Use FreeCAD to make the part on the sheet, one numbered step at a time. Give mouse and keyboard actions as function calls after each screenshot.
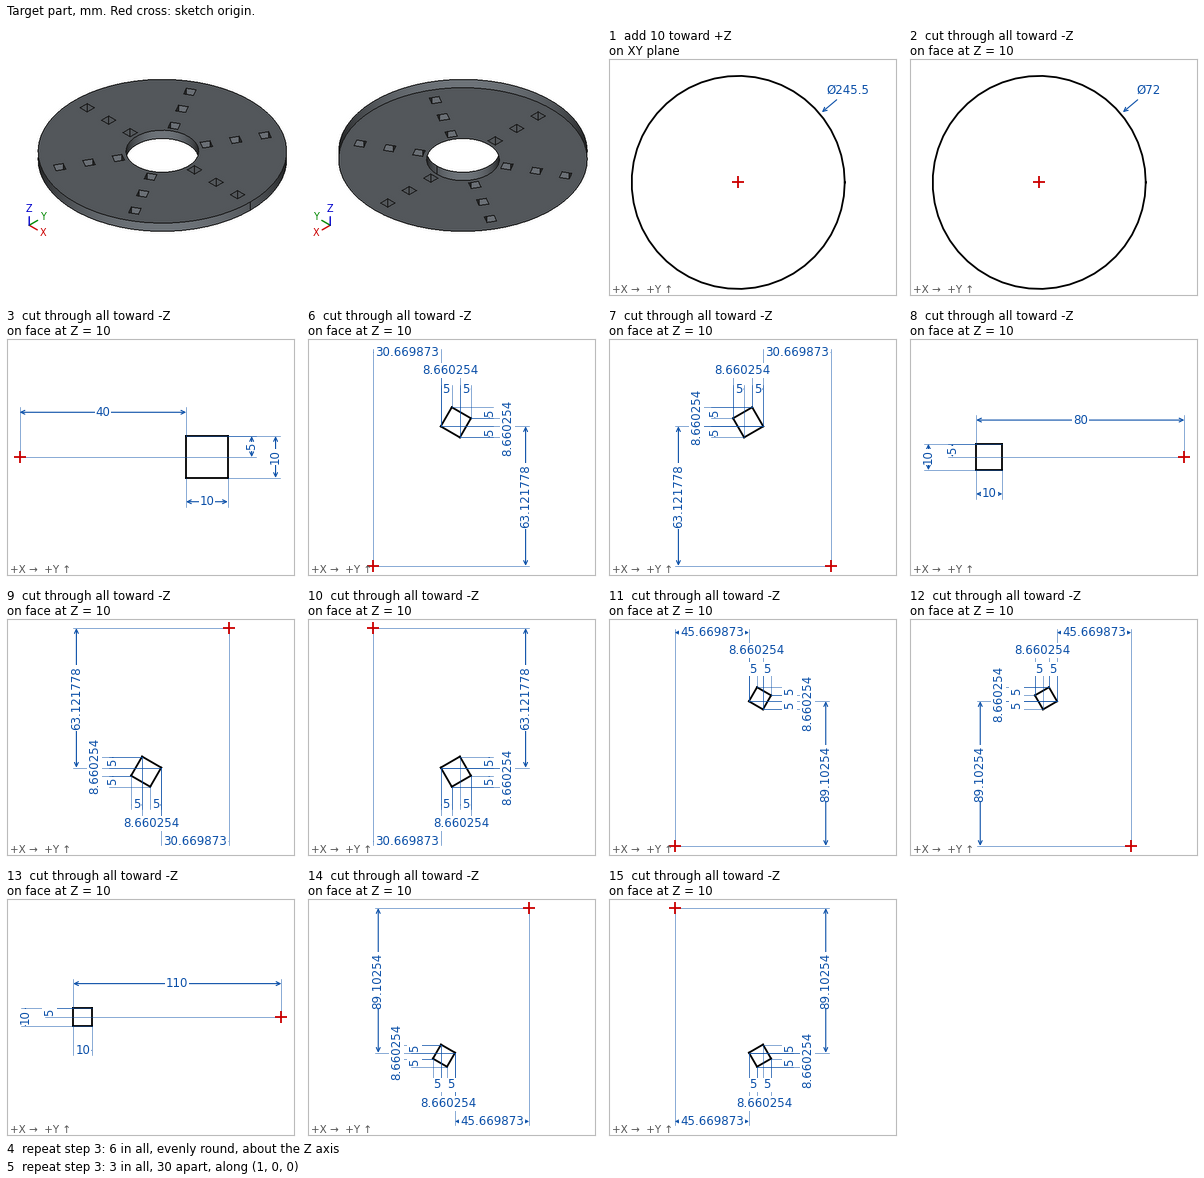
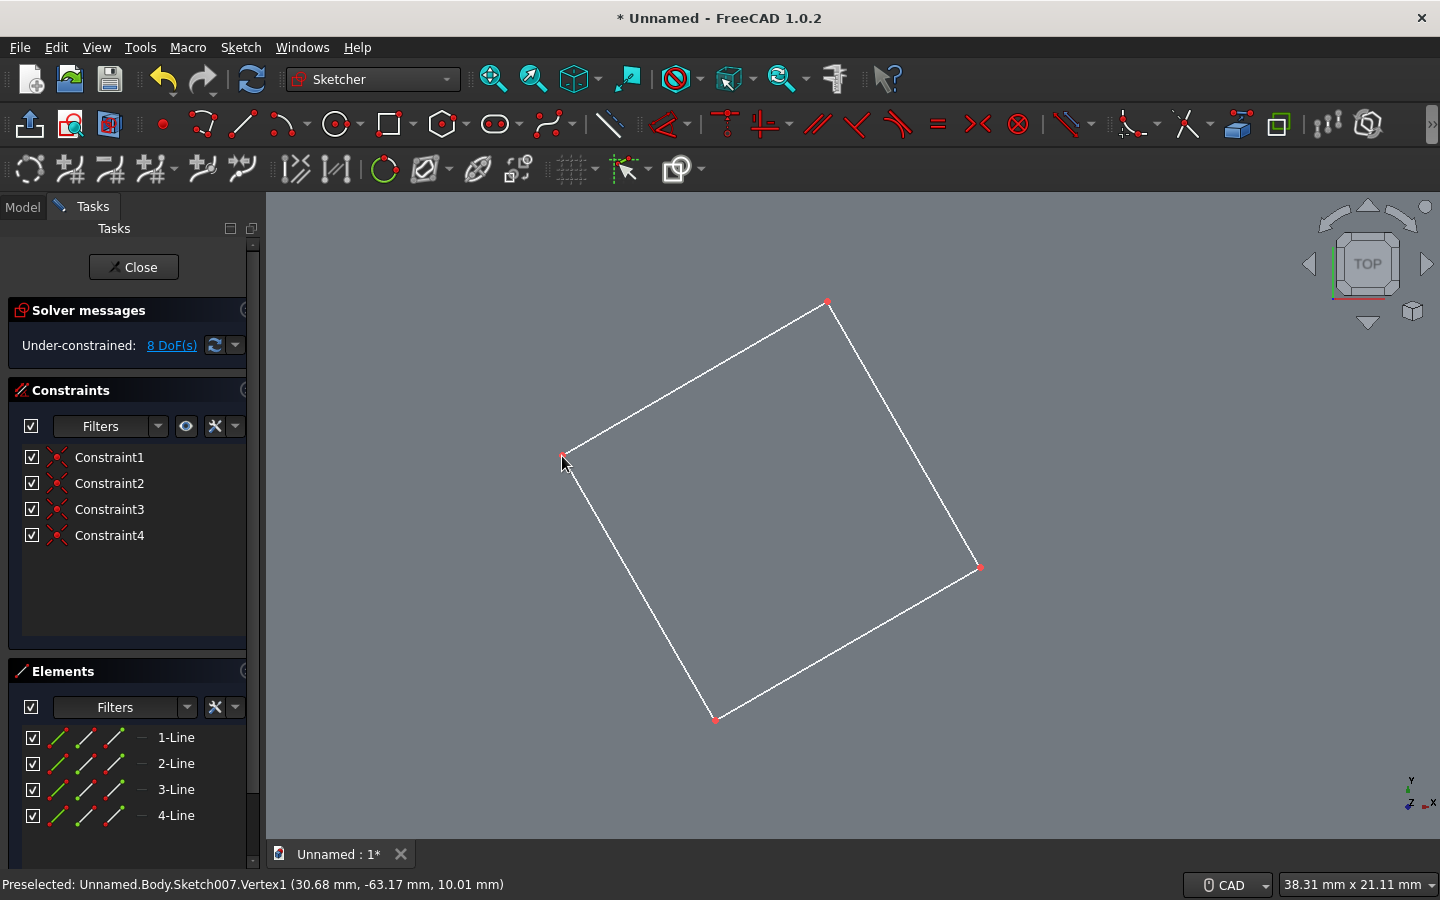
click(664, 124)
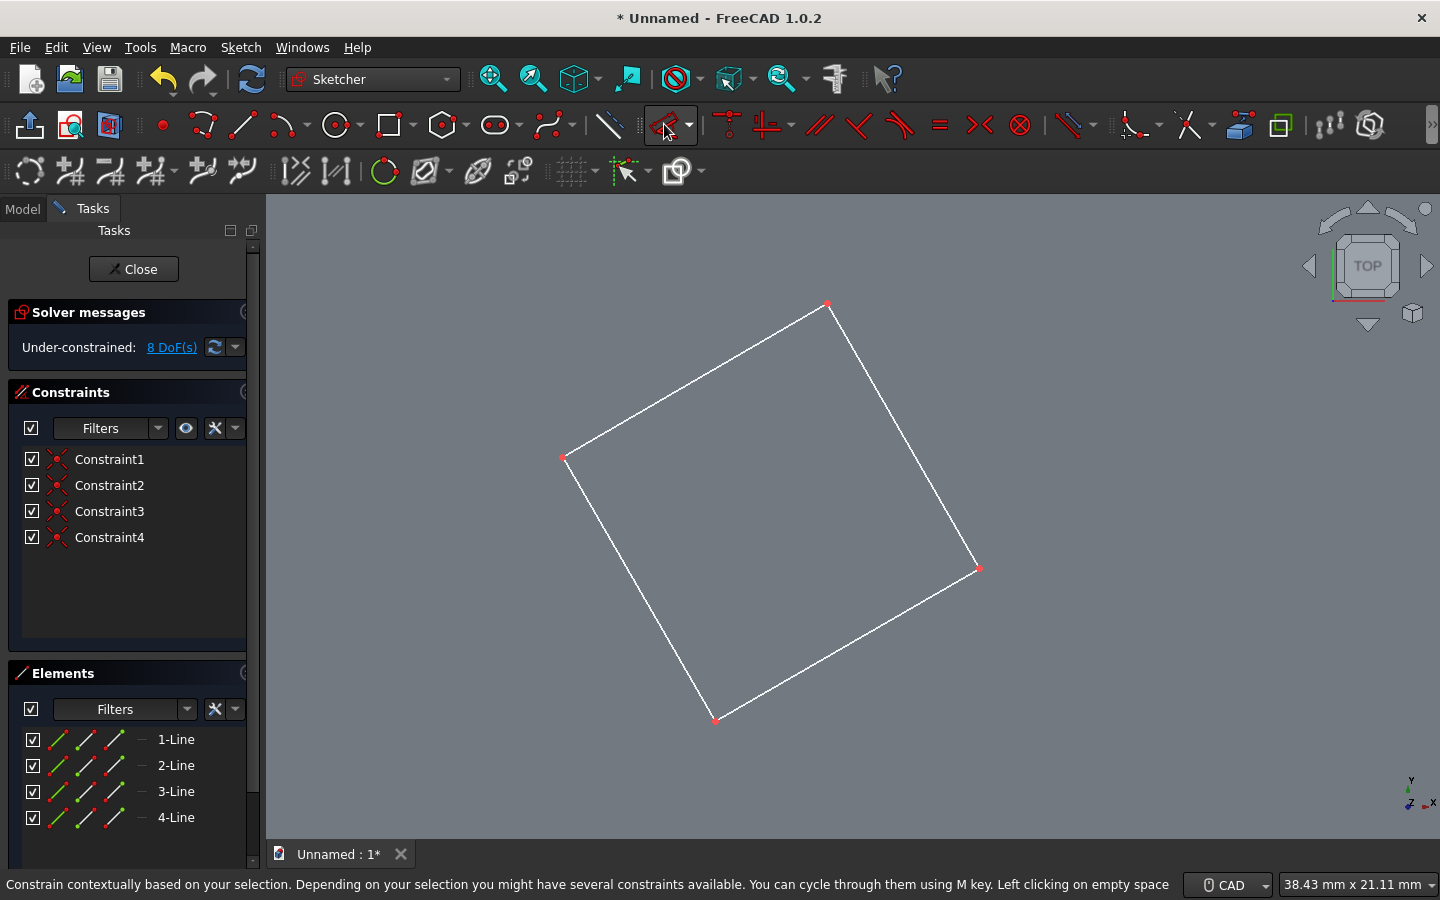
click(609, 536)
click(639, 755)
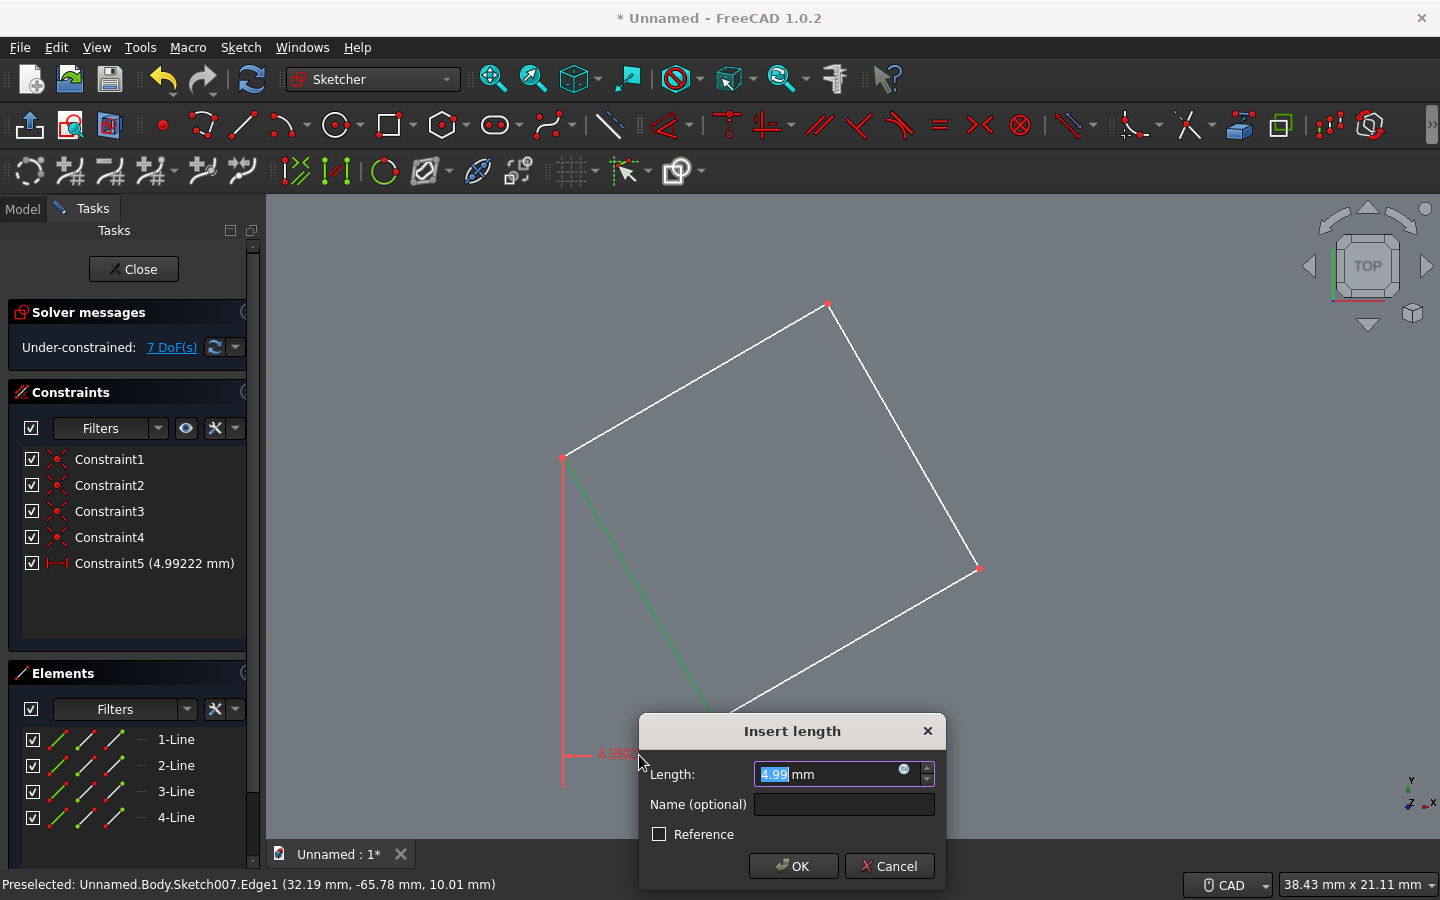
text(5)
key(Return)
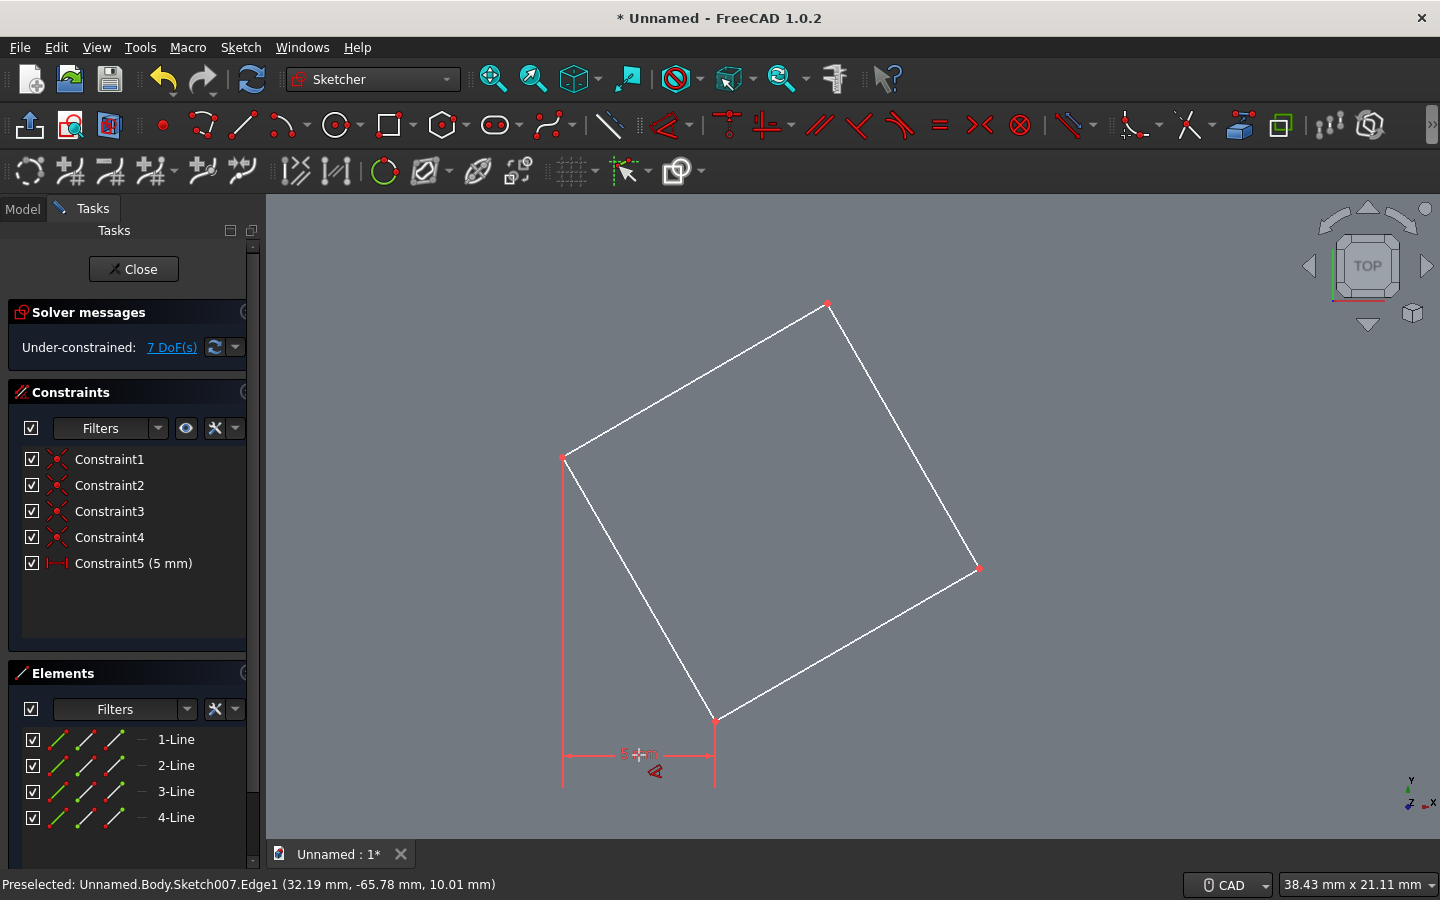
click(795, 676)
click(1014, 645)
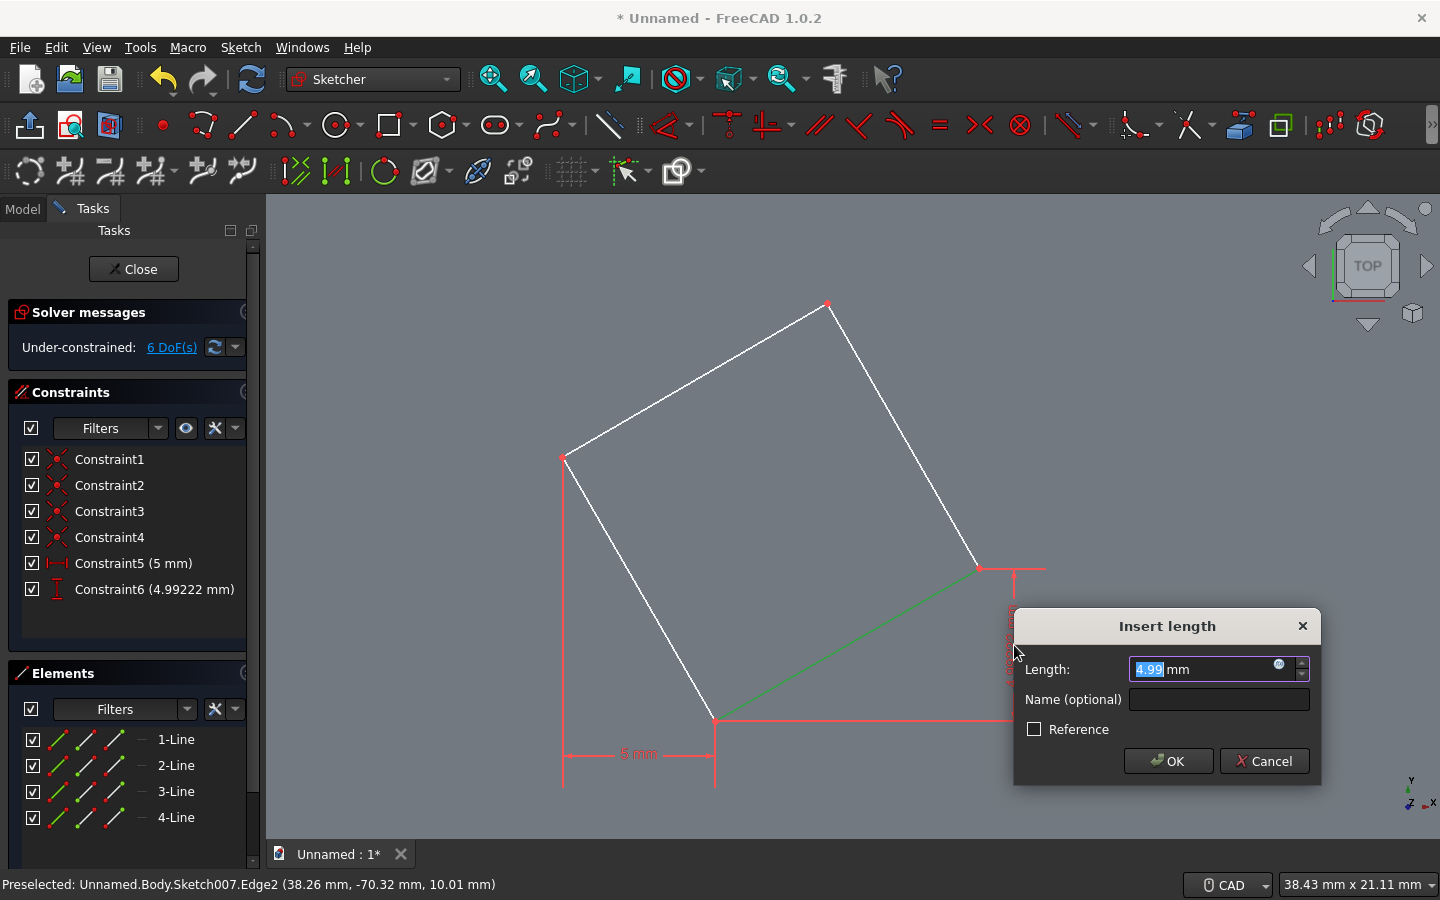
text(5)
key(Return)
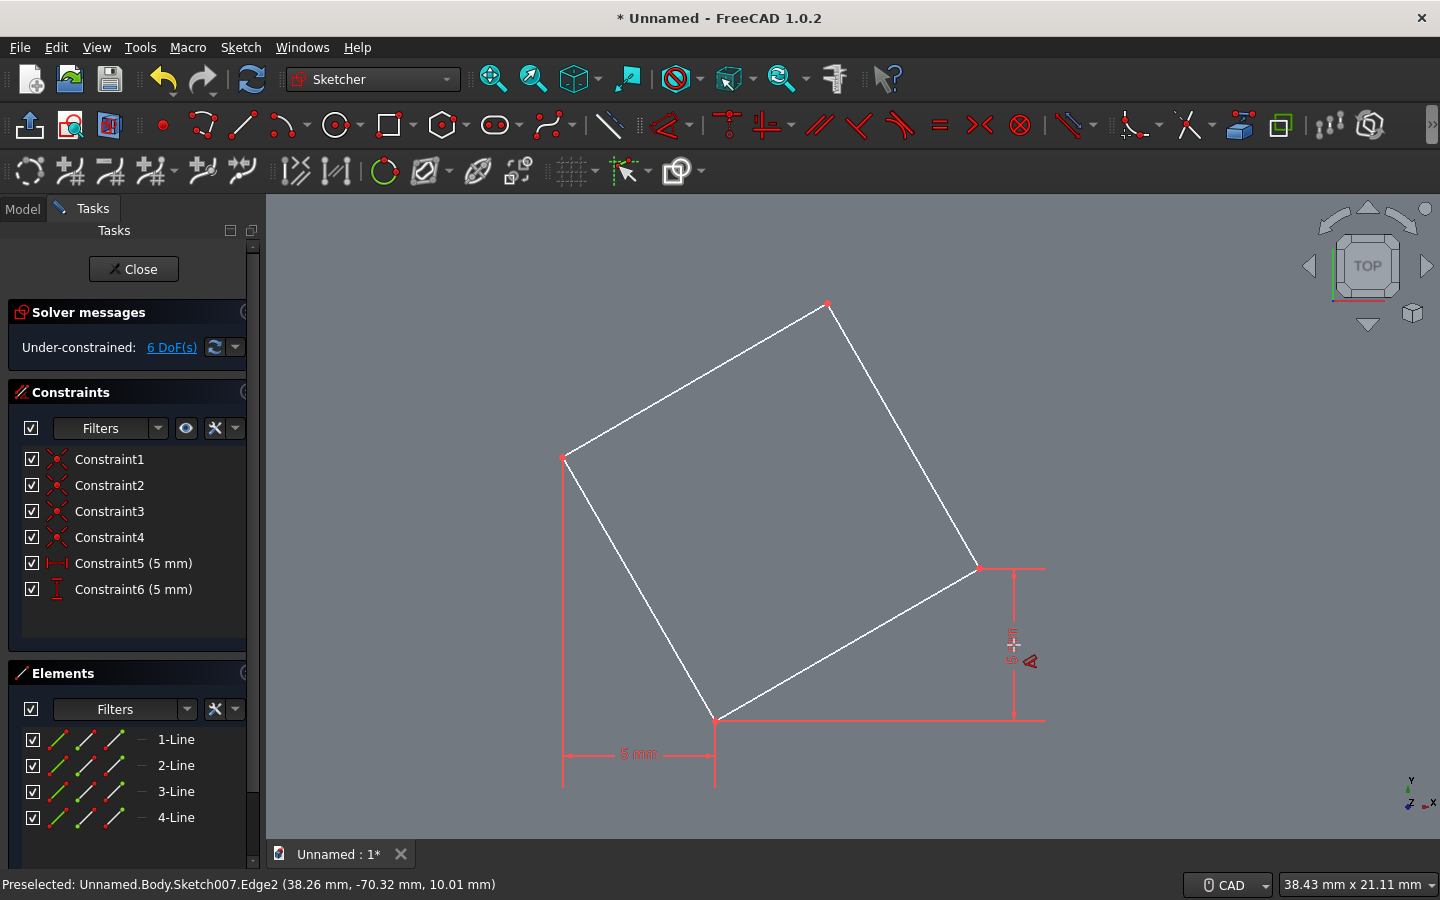
click(934, 489)
click(903, 270)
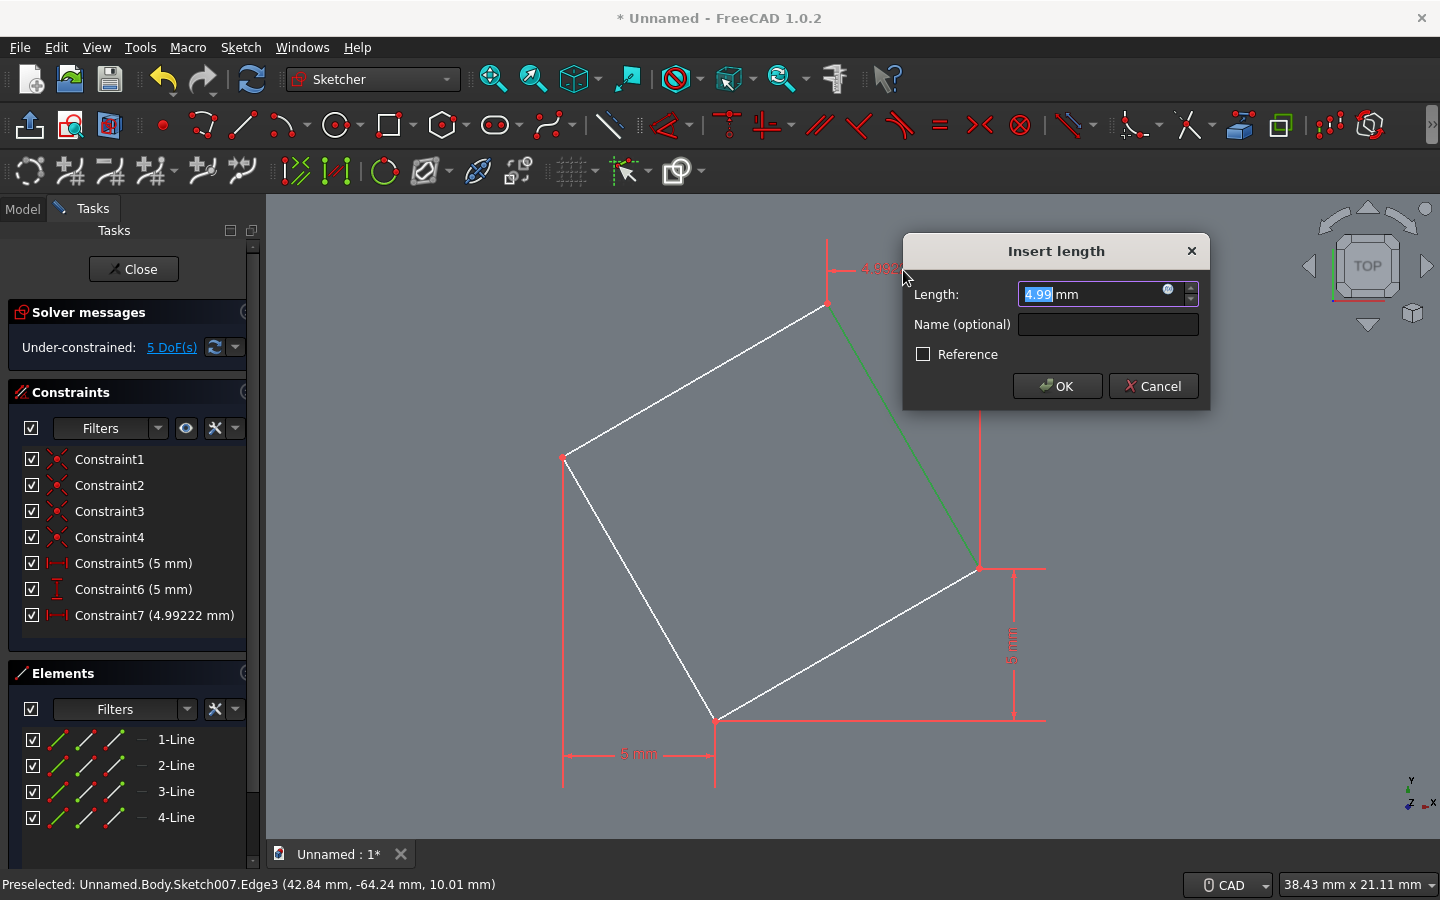
text(5)
key(Return)